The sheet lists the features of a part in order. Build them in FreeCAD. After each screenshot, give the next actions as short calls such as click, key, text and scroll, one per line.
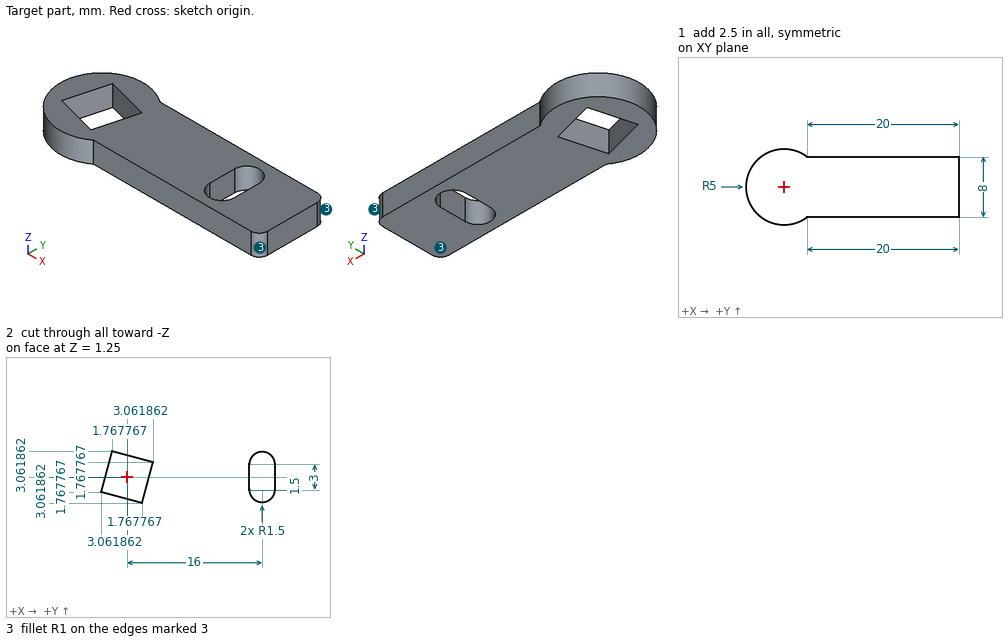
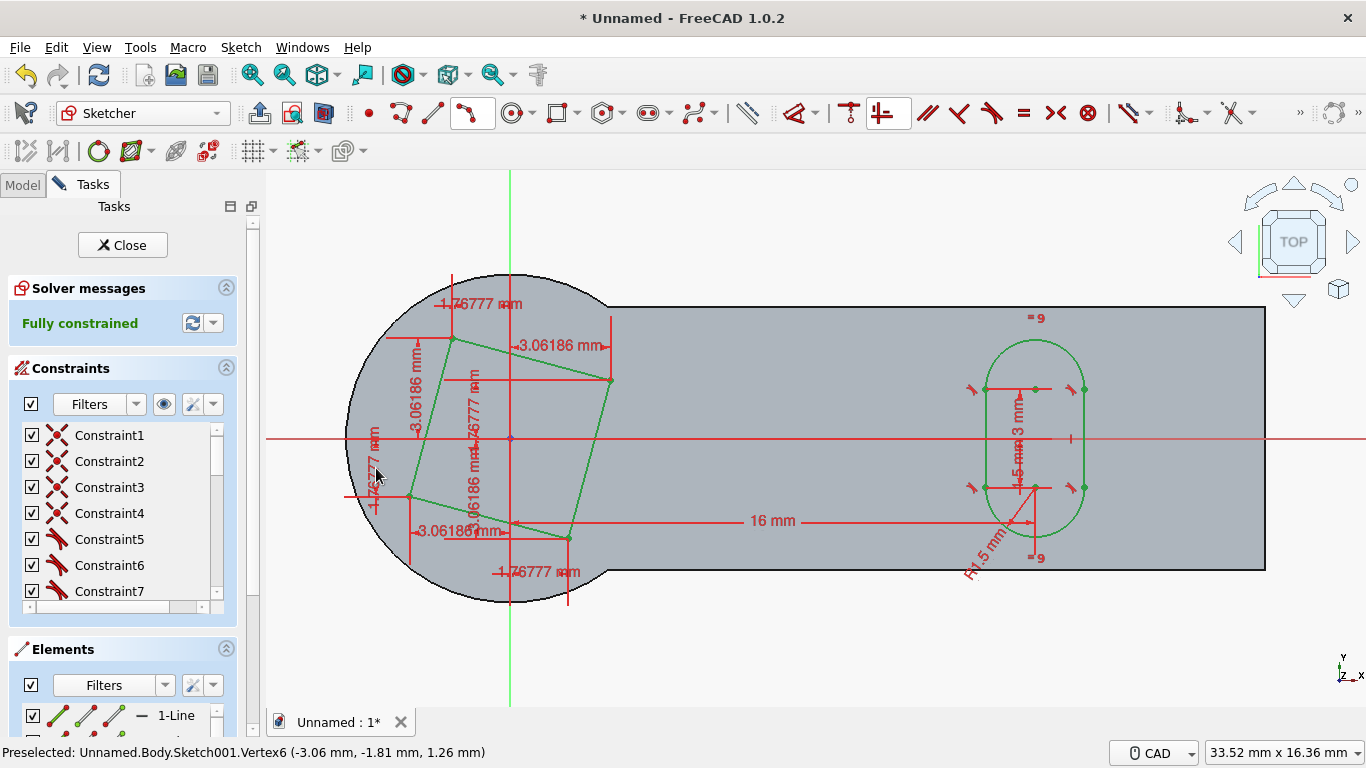
click(123, 245)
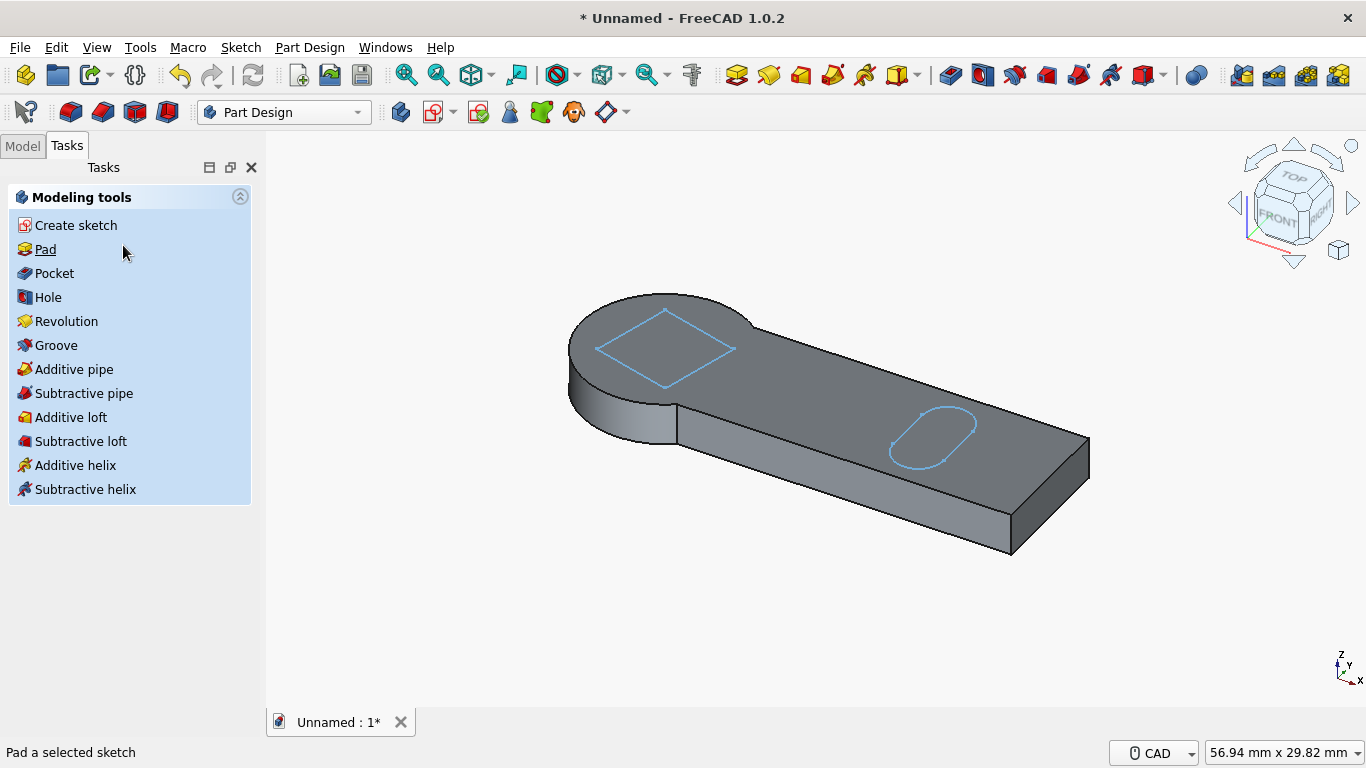
click(952, 76)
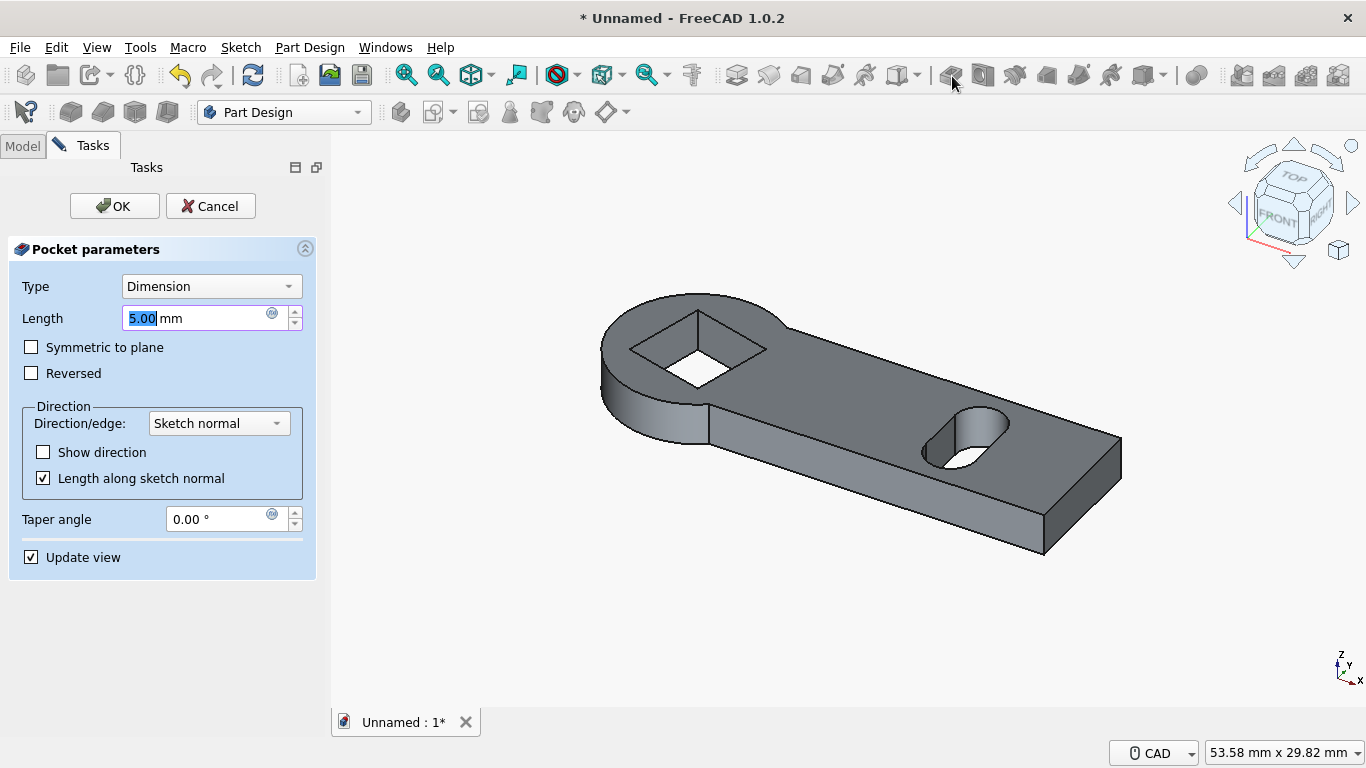
click(212, 286)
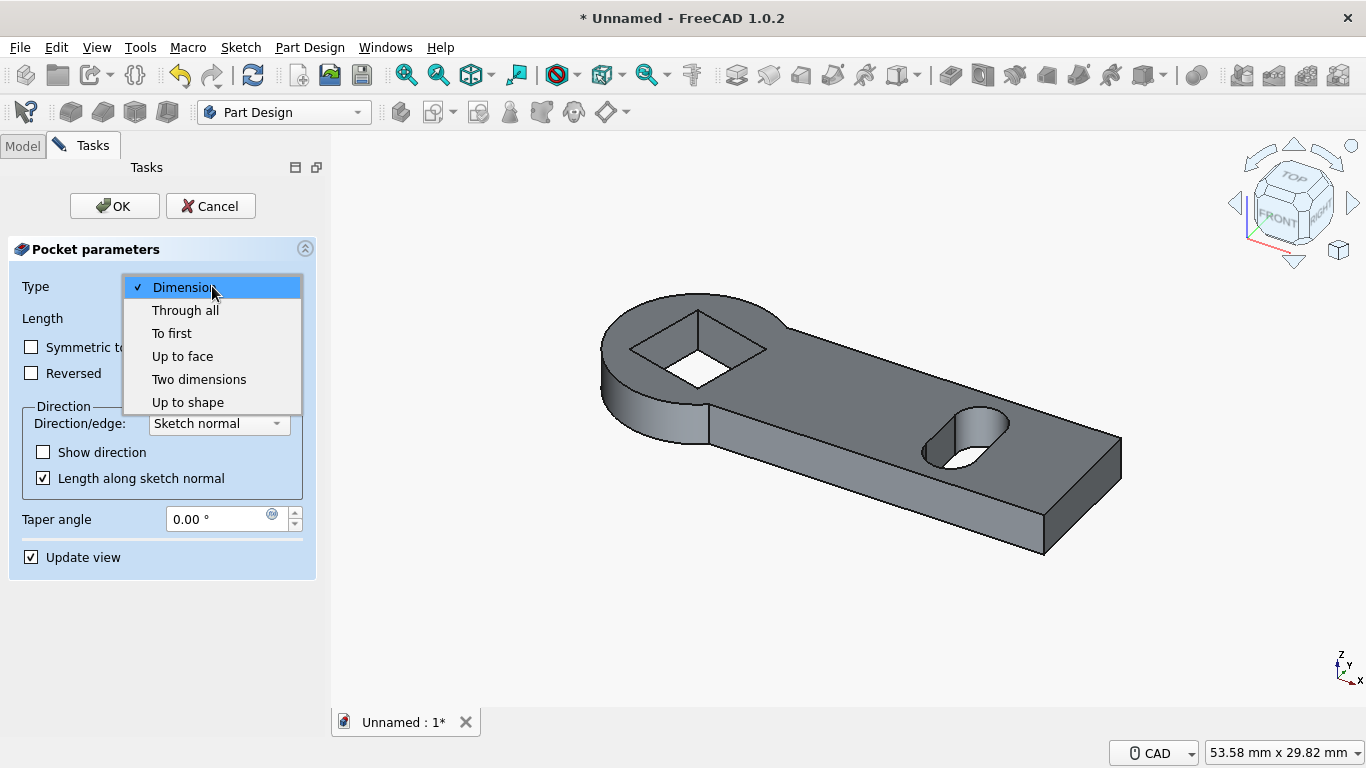
click(212, 310)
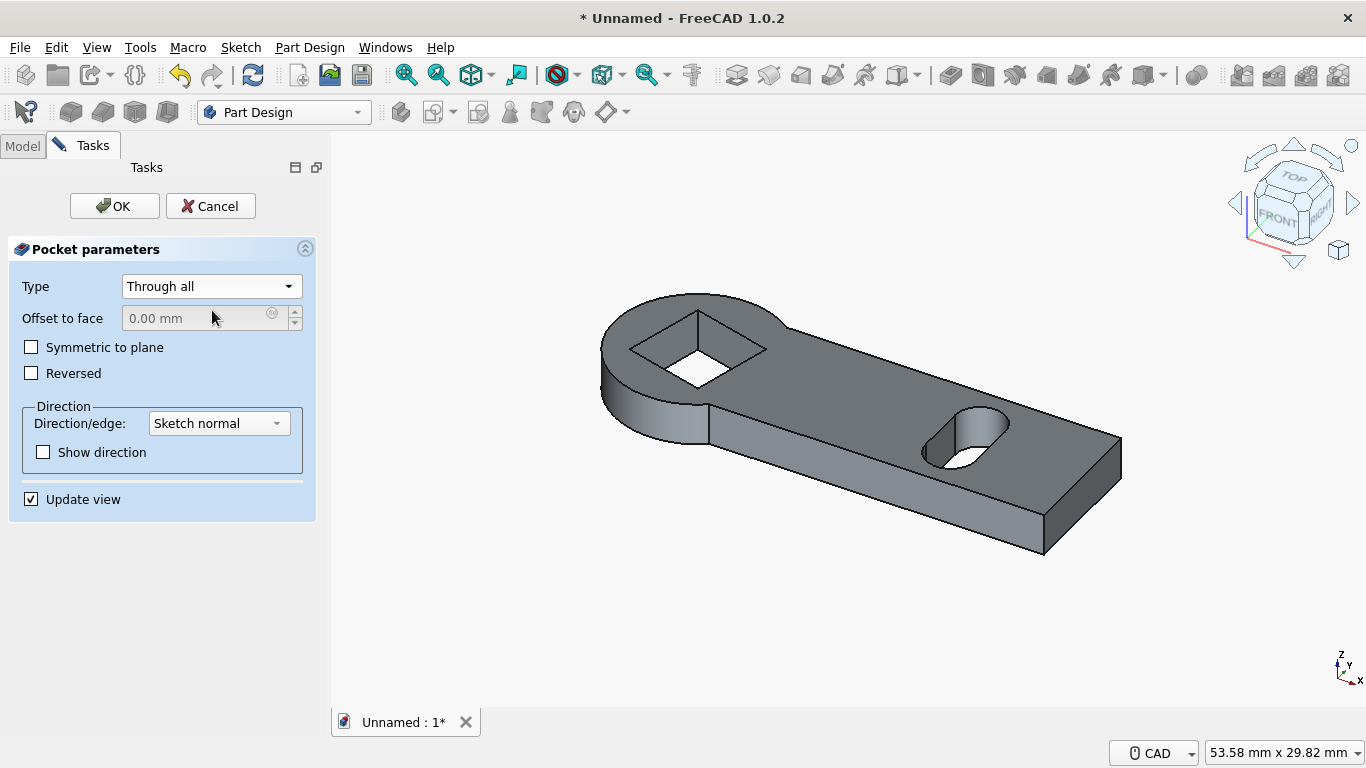
click(115, 206)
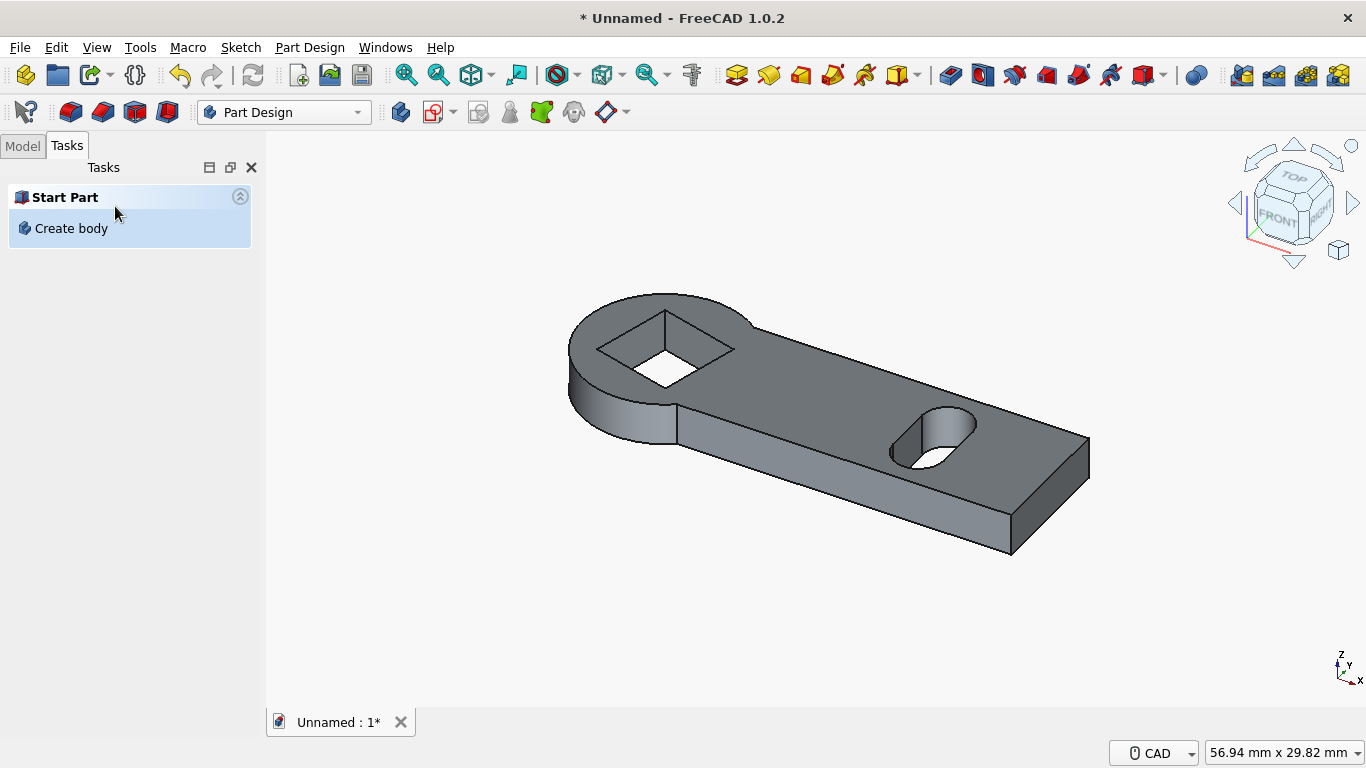
click(1011, 534)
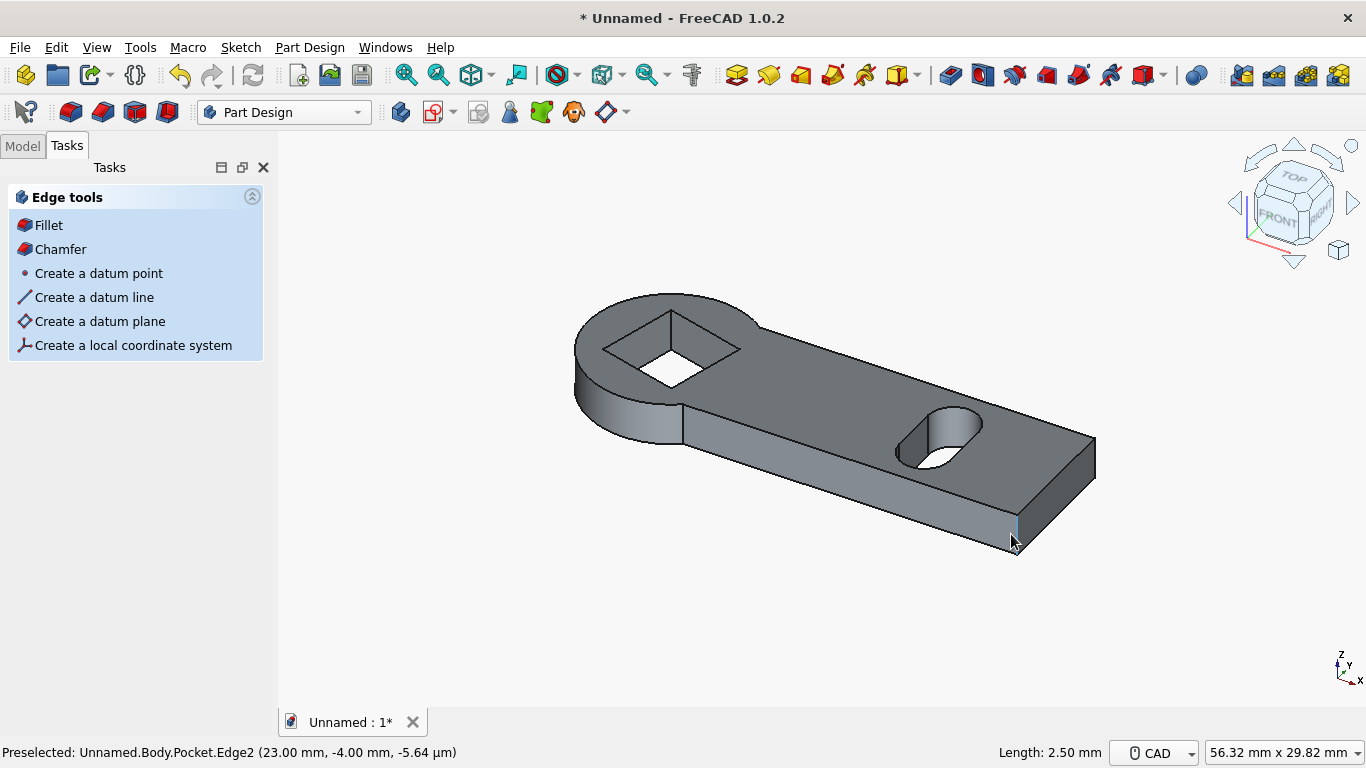
key(0)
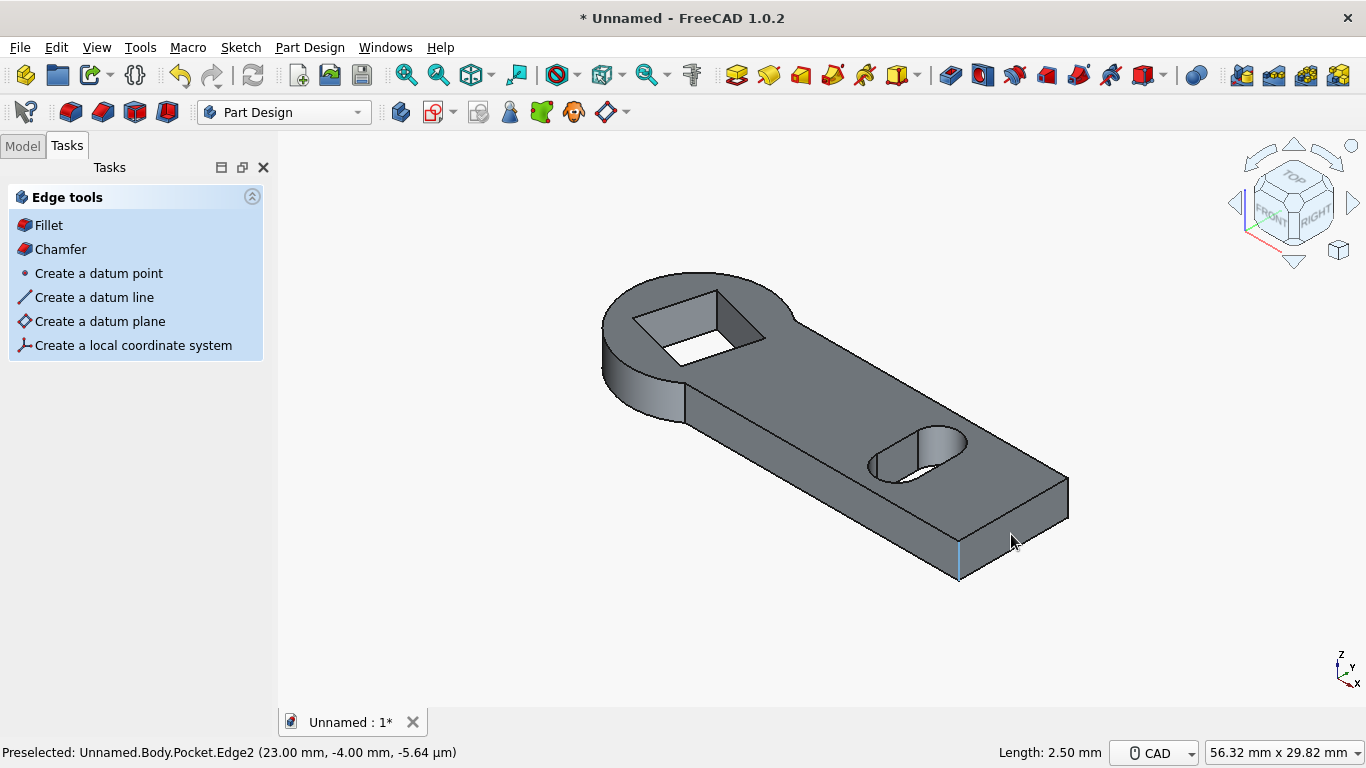
key(2)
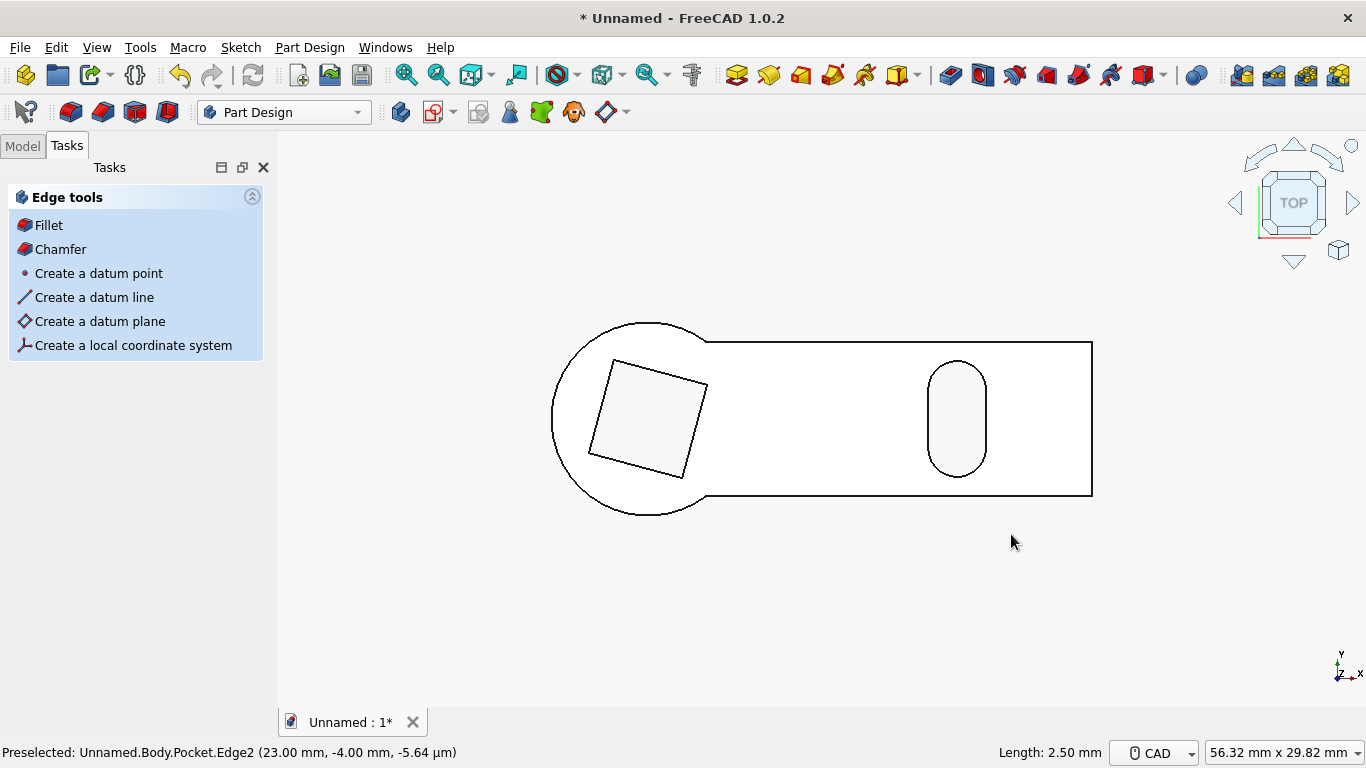
key(1)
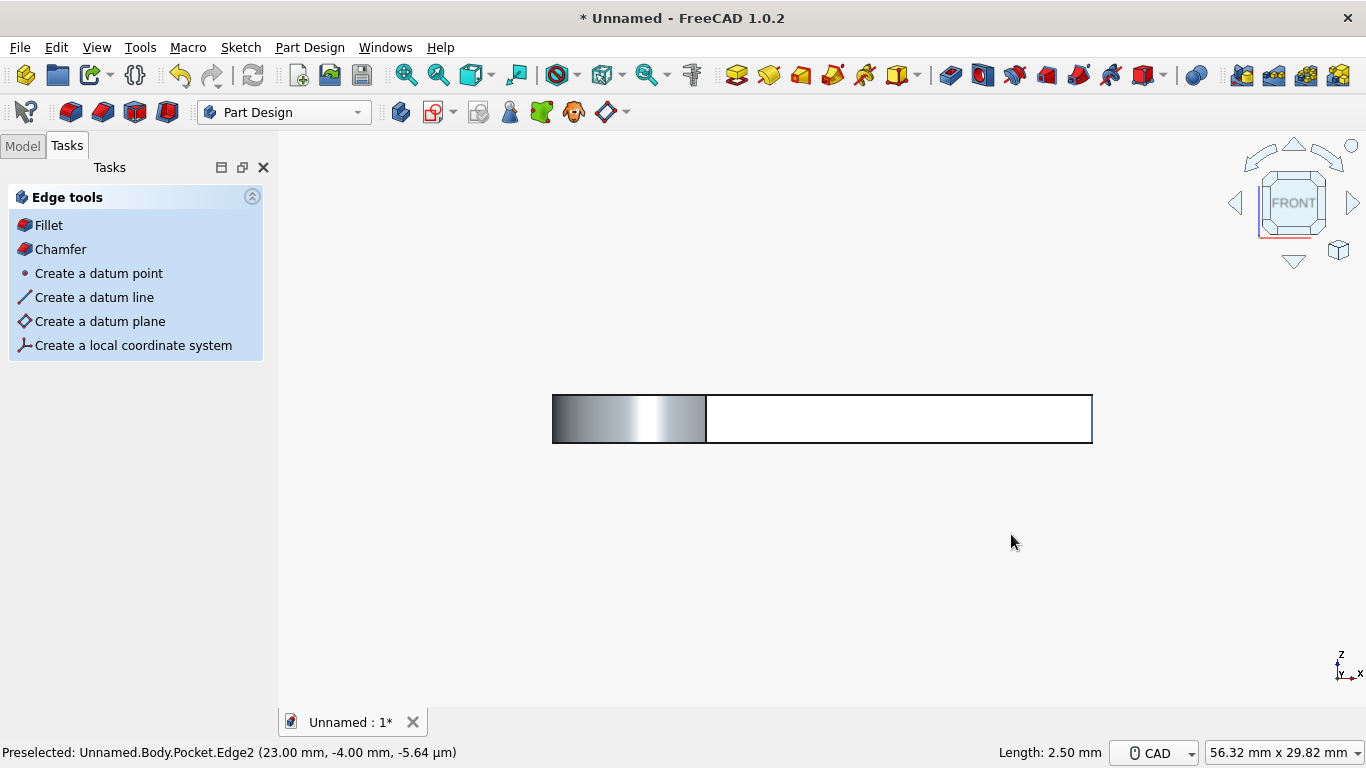
key(3)